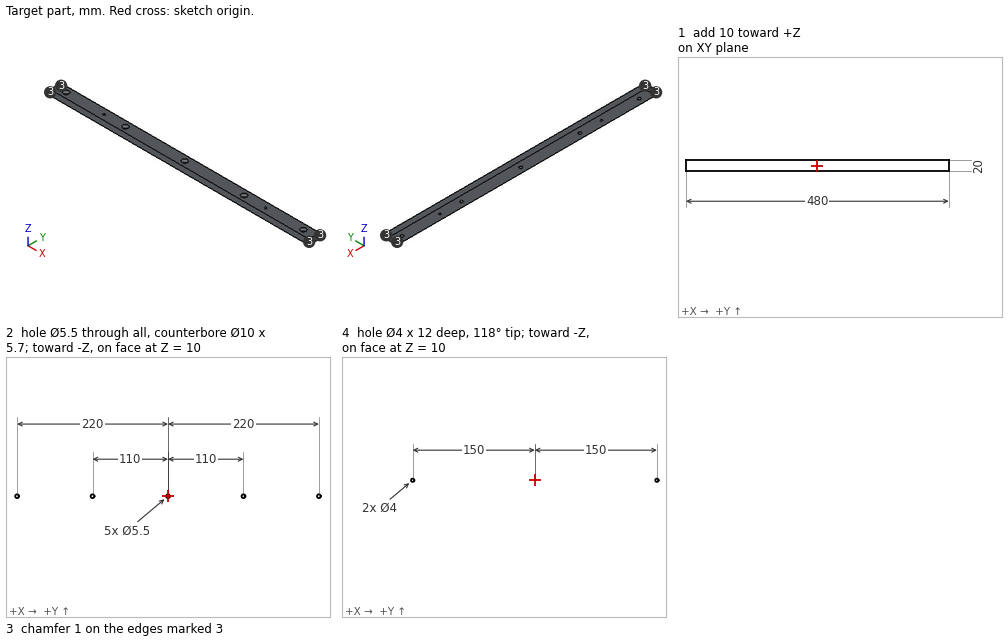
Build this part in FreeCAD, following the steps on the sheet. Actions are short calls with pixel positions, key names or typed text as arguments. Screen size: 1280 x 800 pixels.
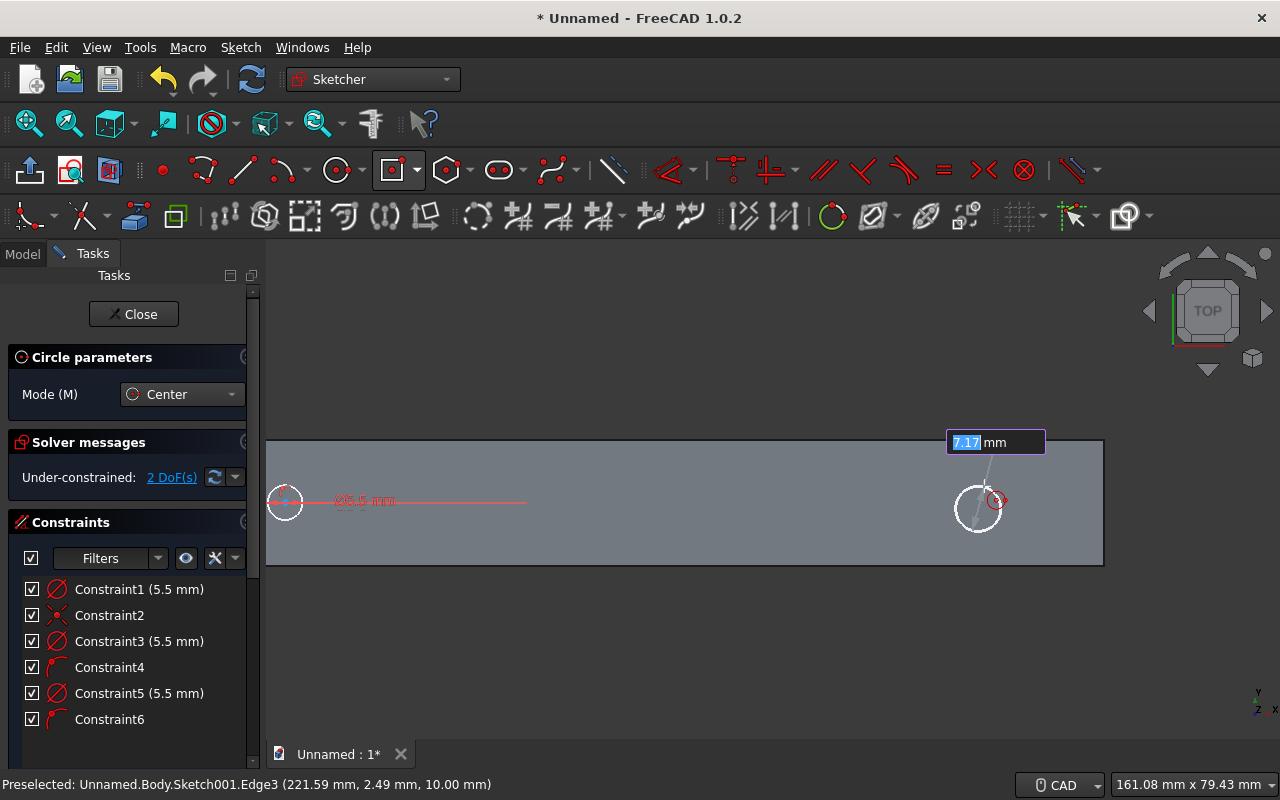
text(5.5)
key(Return)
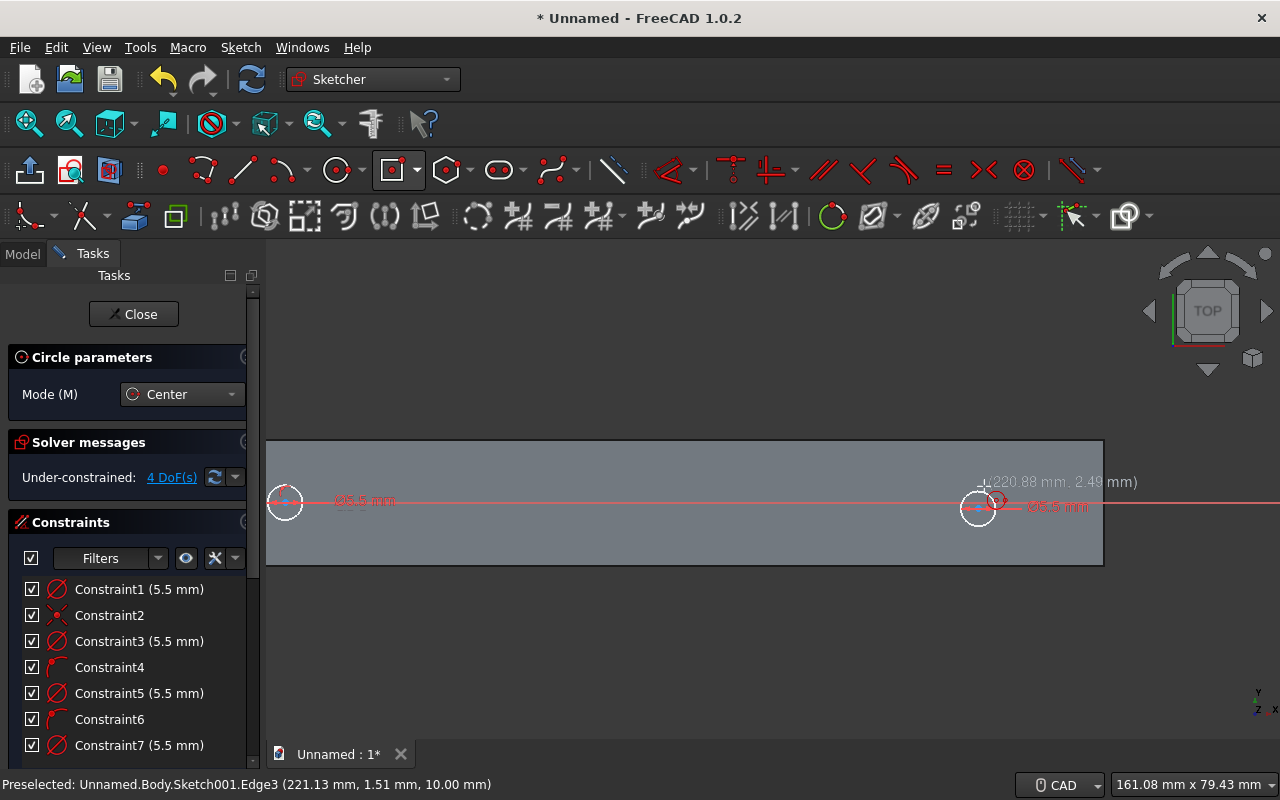
scroll(986, 486, down, 8)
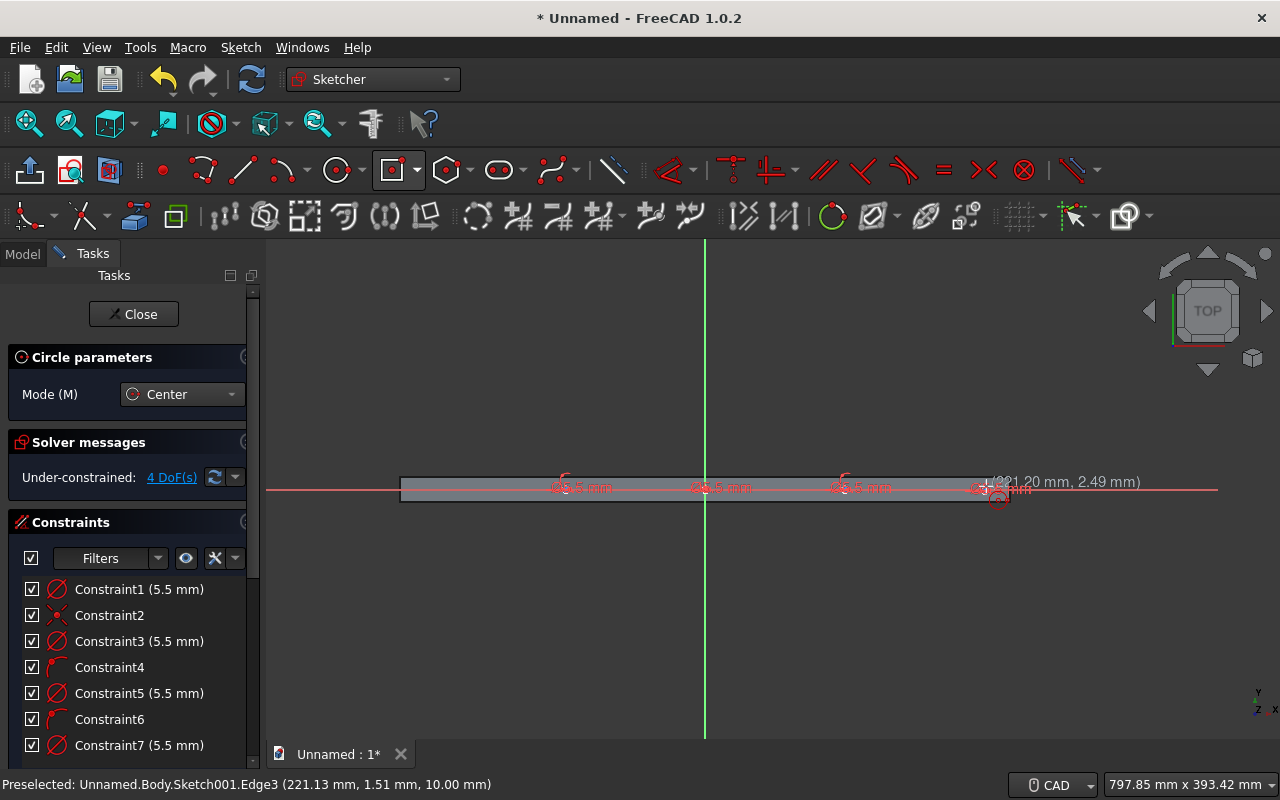
scroll(426, 490, up, 10)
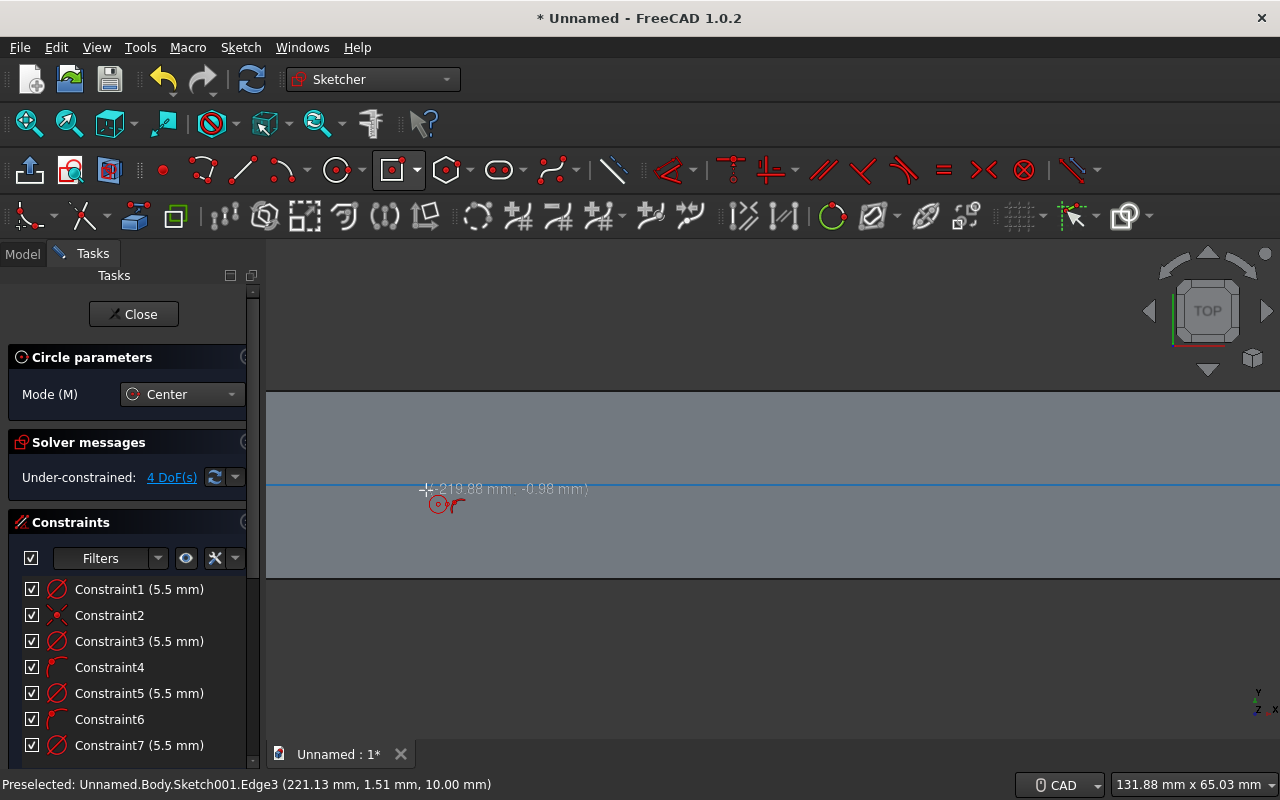
scroll(425, 490, down, 10)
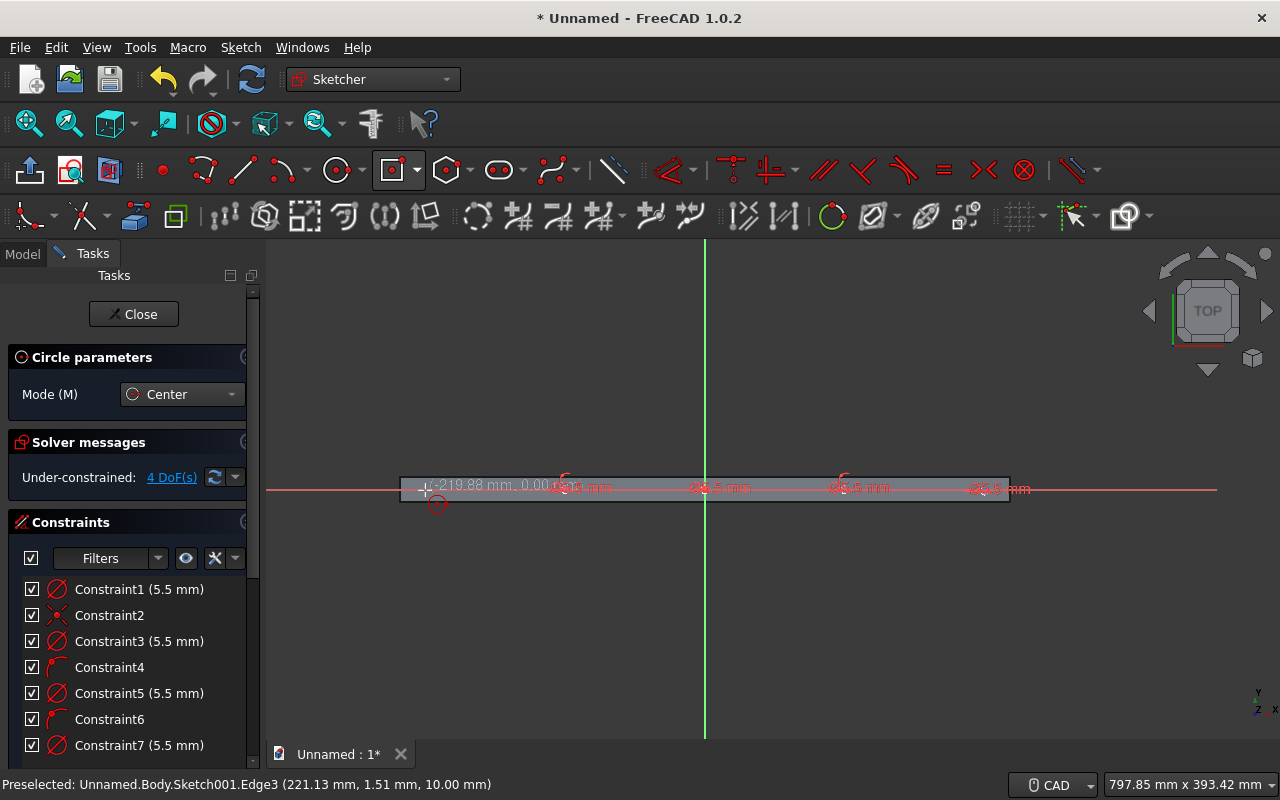
click(425, 490)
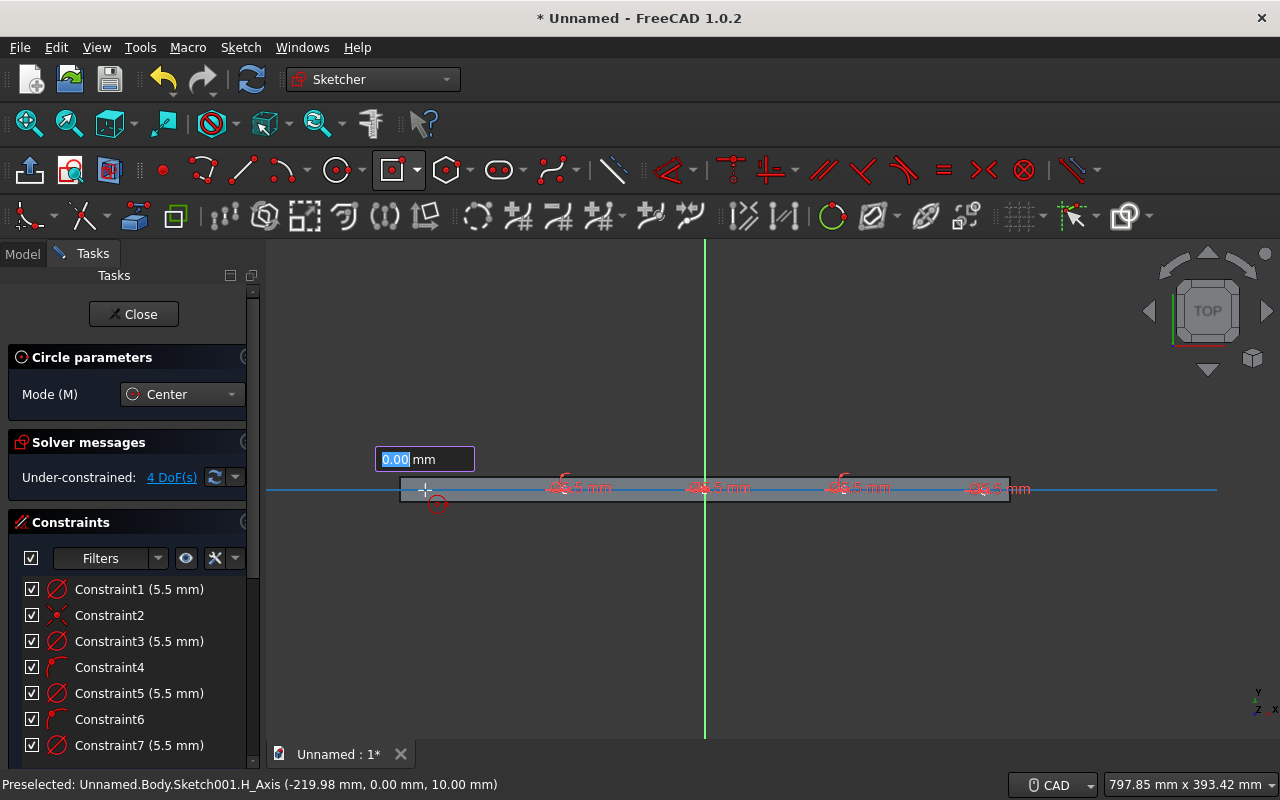
scroll(426, 486, up, 8)
move(426, 486)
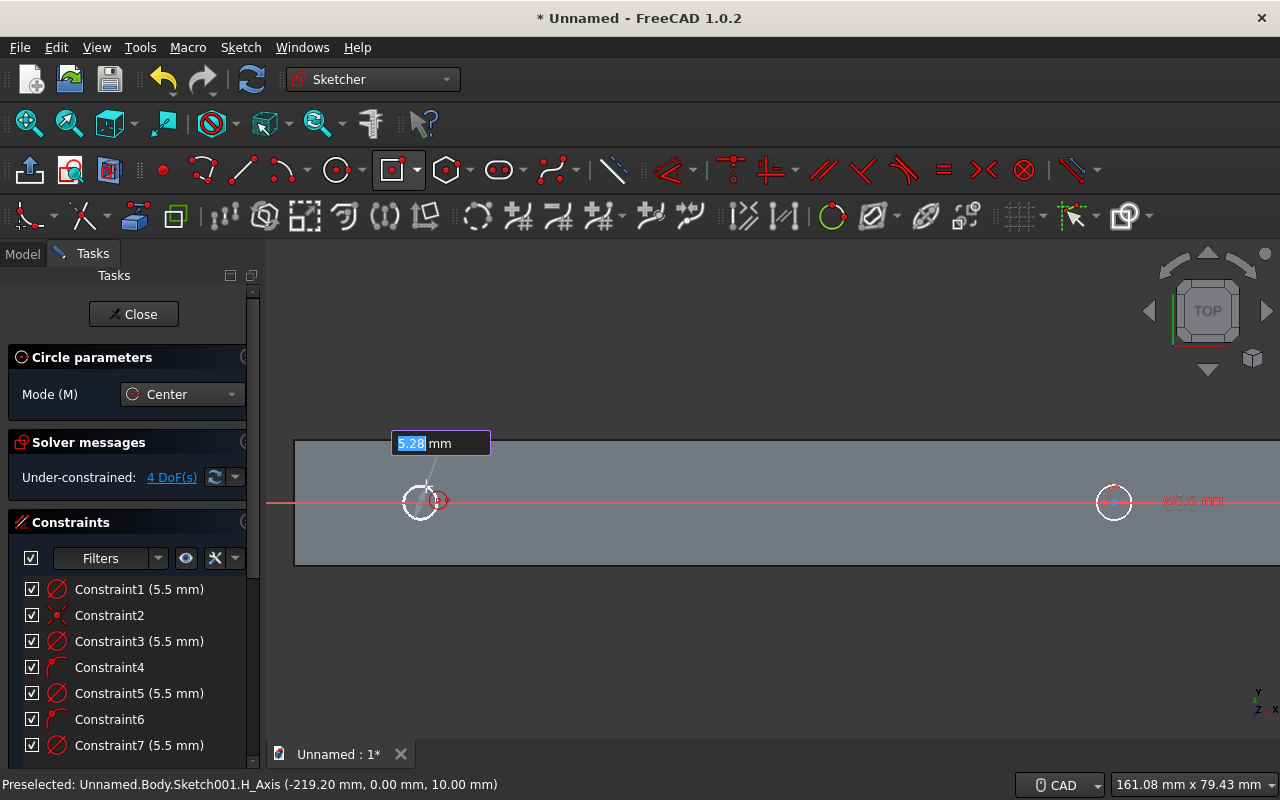
text(5.5)
key(Return)
key(Escape)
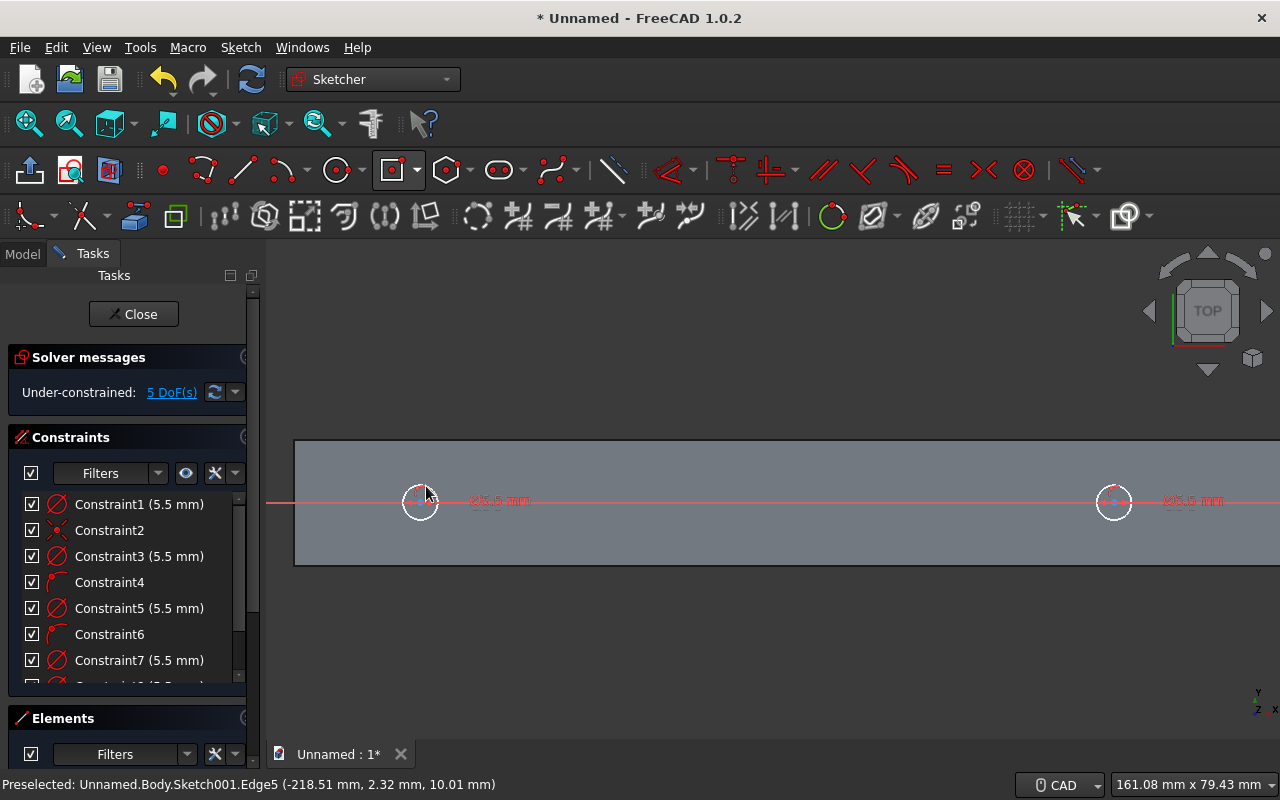
scroll(426, 486, down, 8)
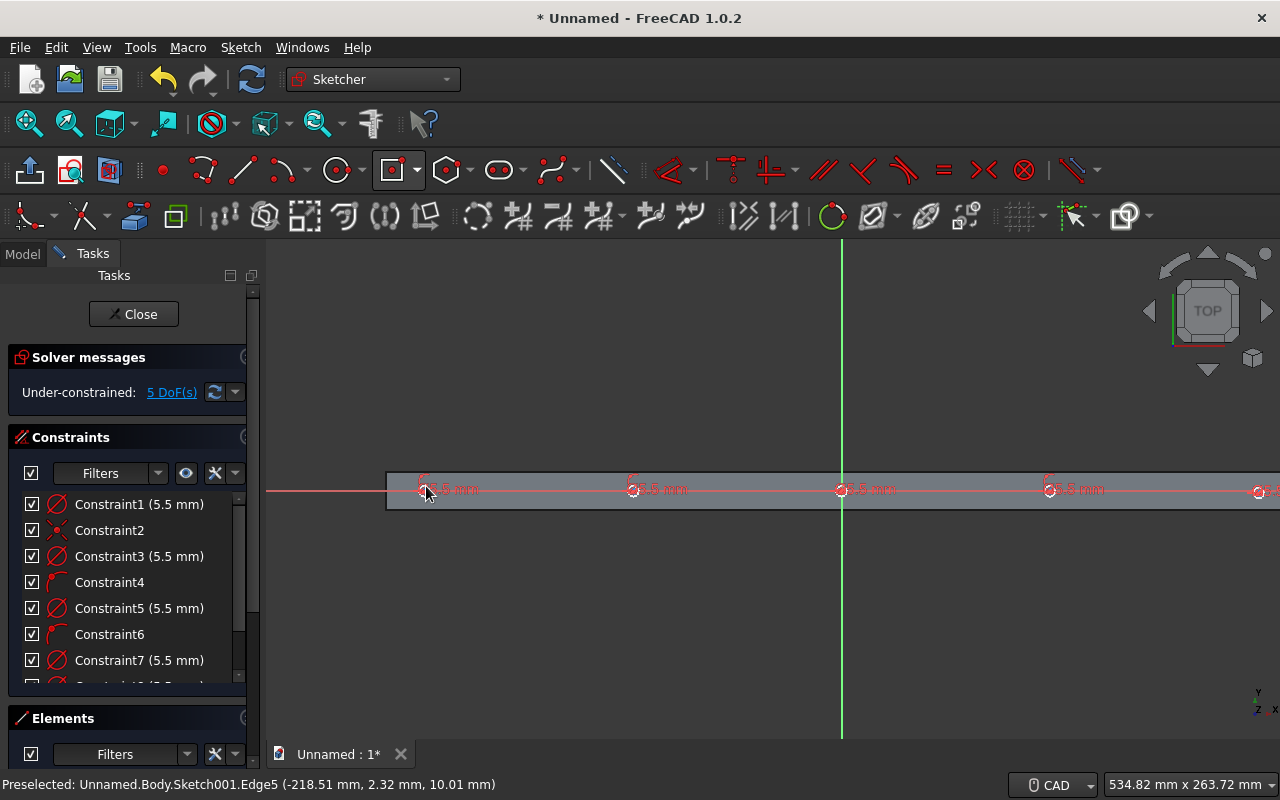
click(984, 491)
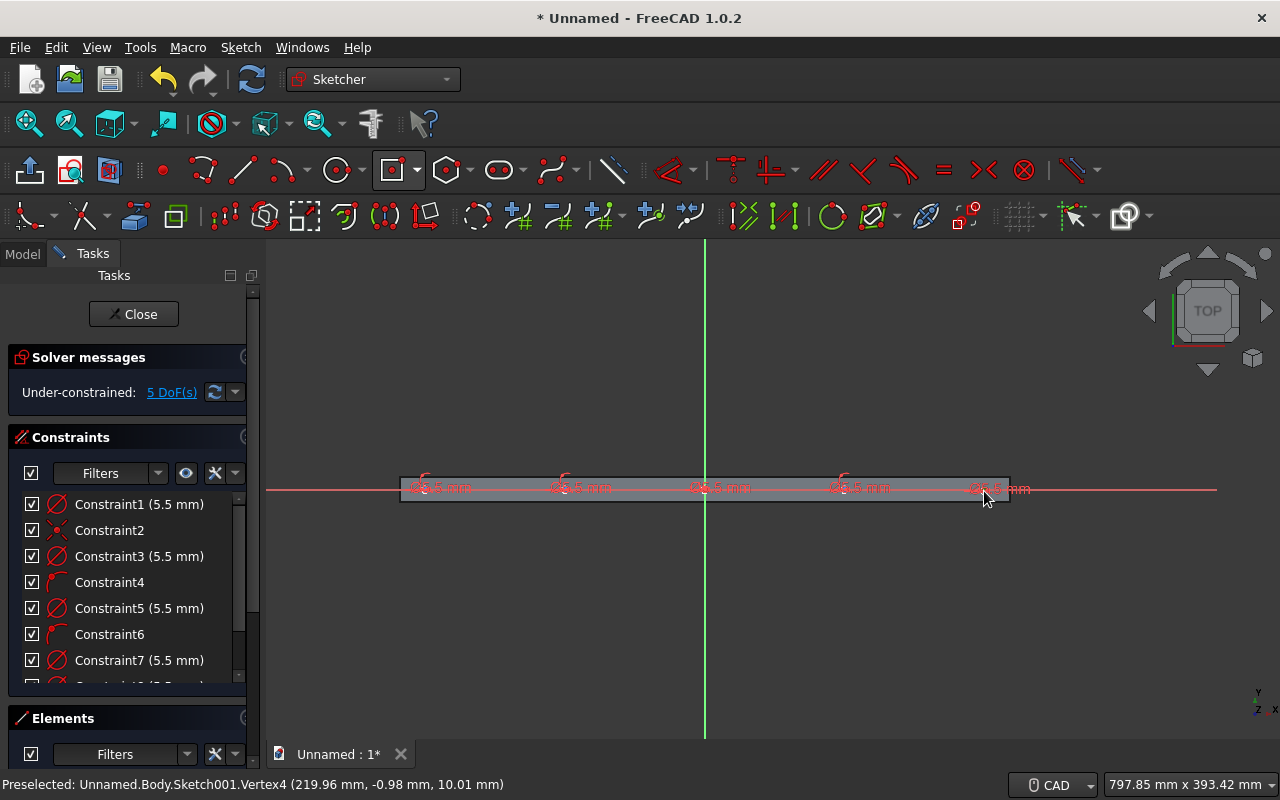
click(353, 490)